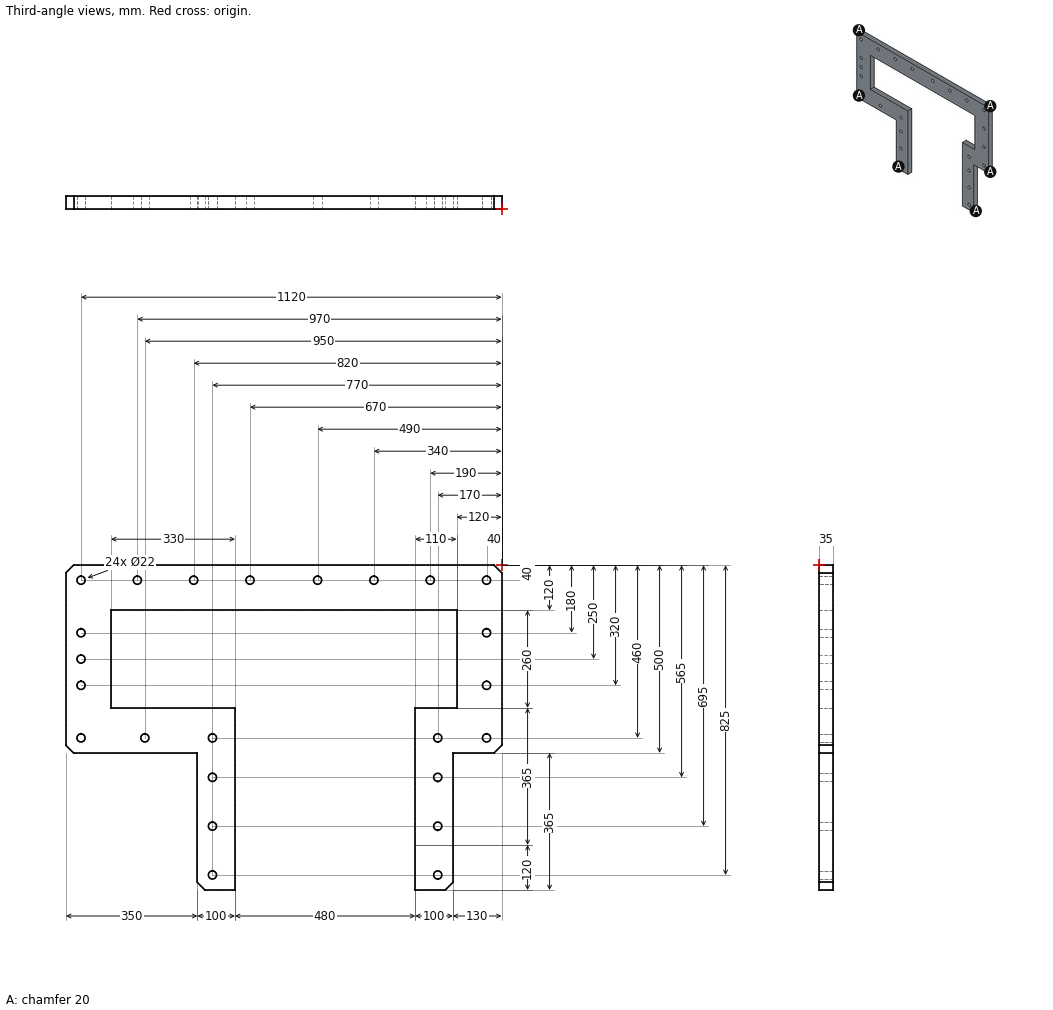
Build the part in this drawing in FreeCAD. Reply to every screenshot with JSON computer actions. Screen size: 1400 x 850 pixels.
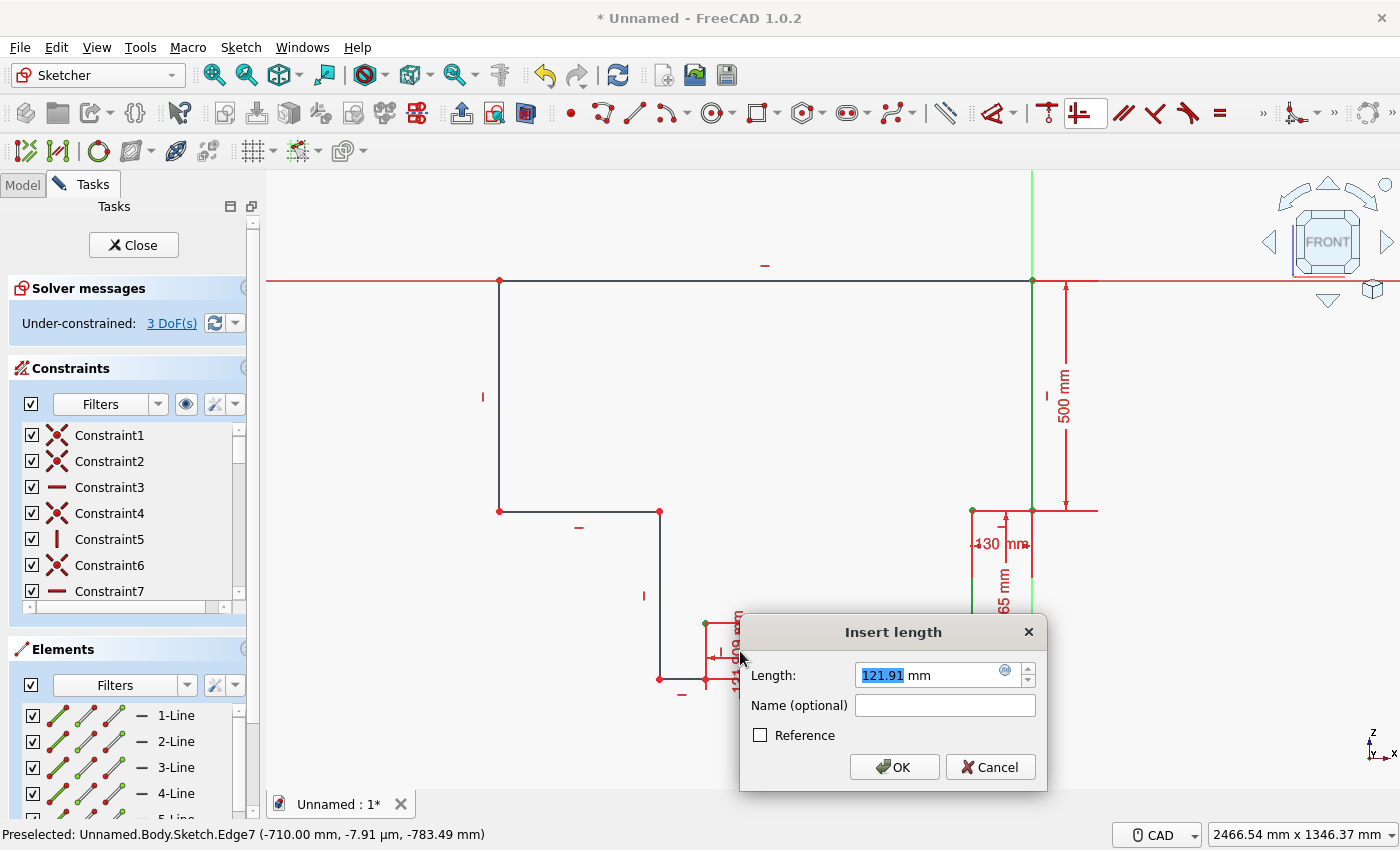
{"action": "type", "text": "120"}
{"action": "key", "text": "Return"}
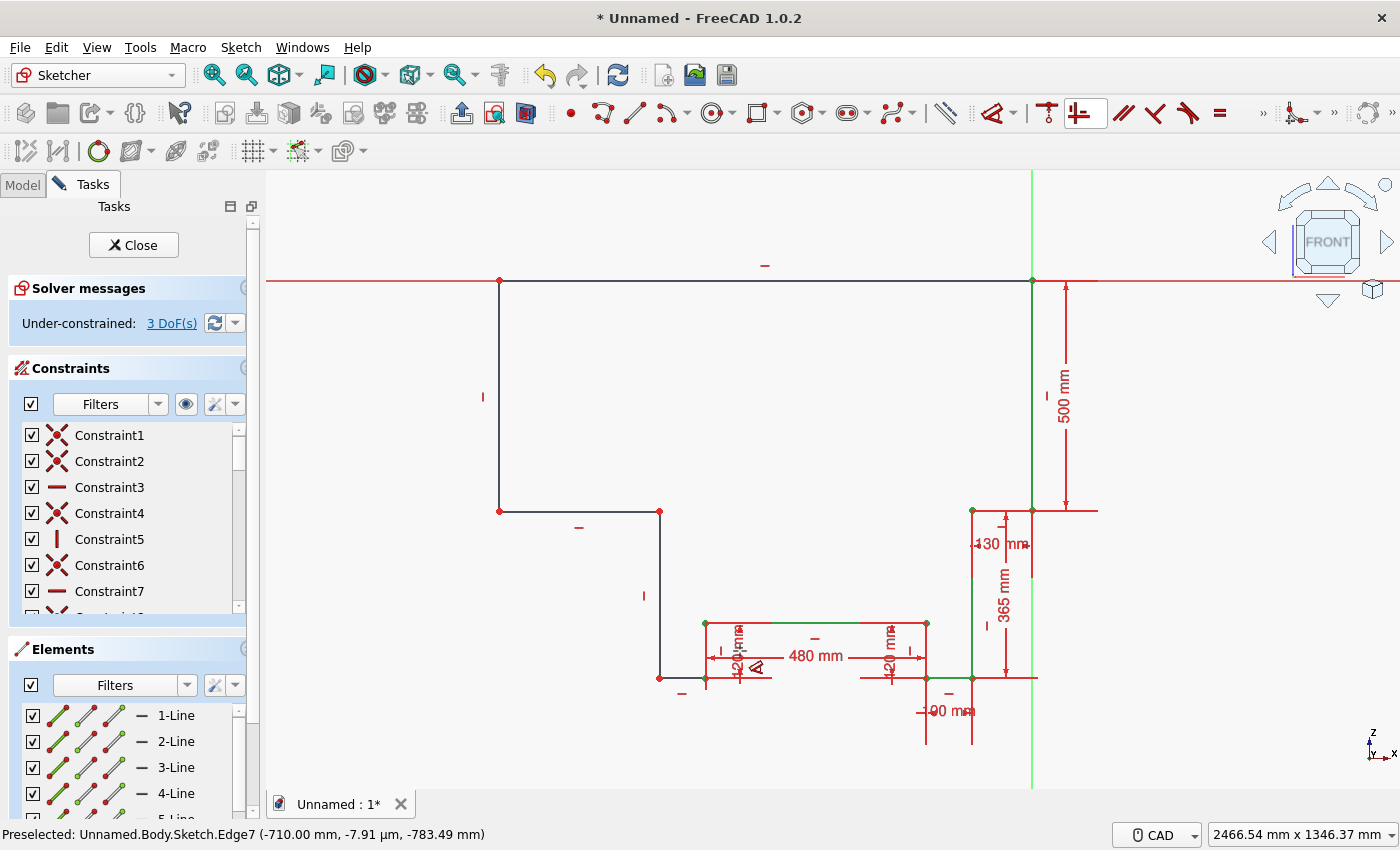
{"action": "left_click", "coordinate": [692, 678]}
{"action": "left_click", "coordinate": [683, 712]}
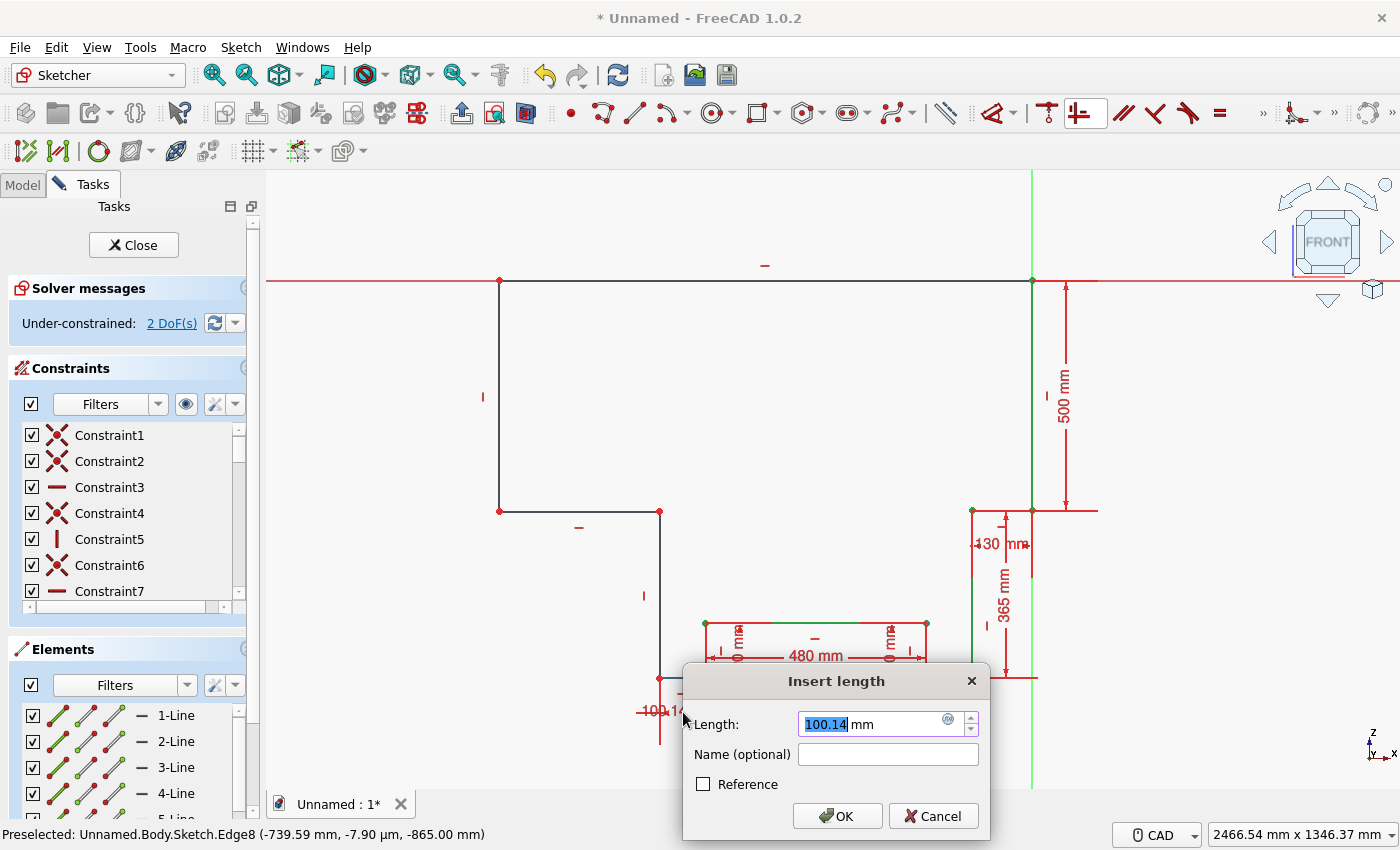
{"action": "type", "text": "100"}
{"action": "key", "text": "Return"}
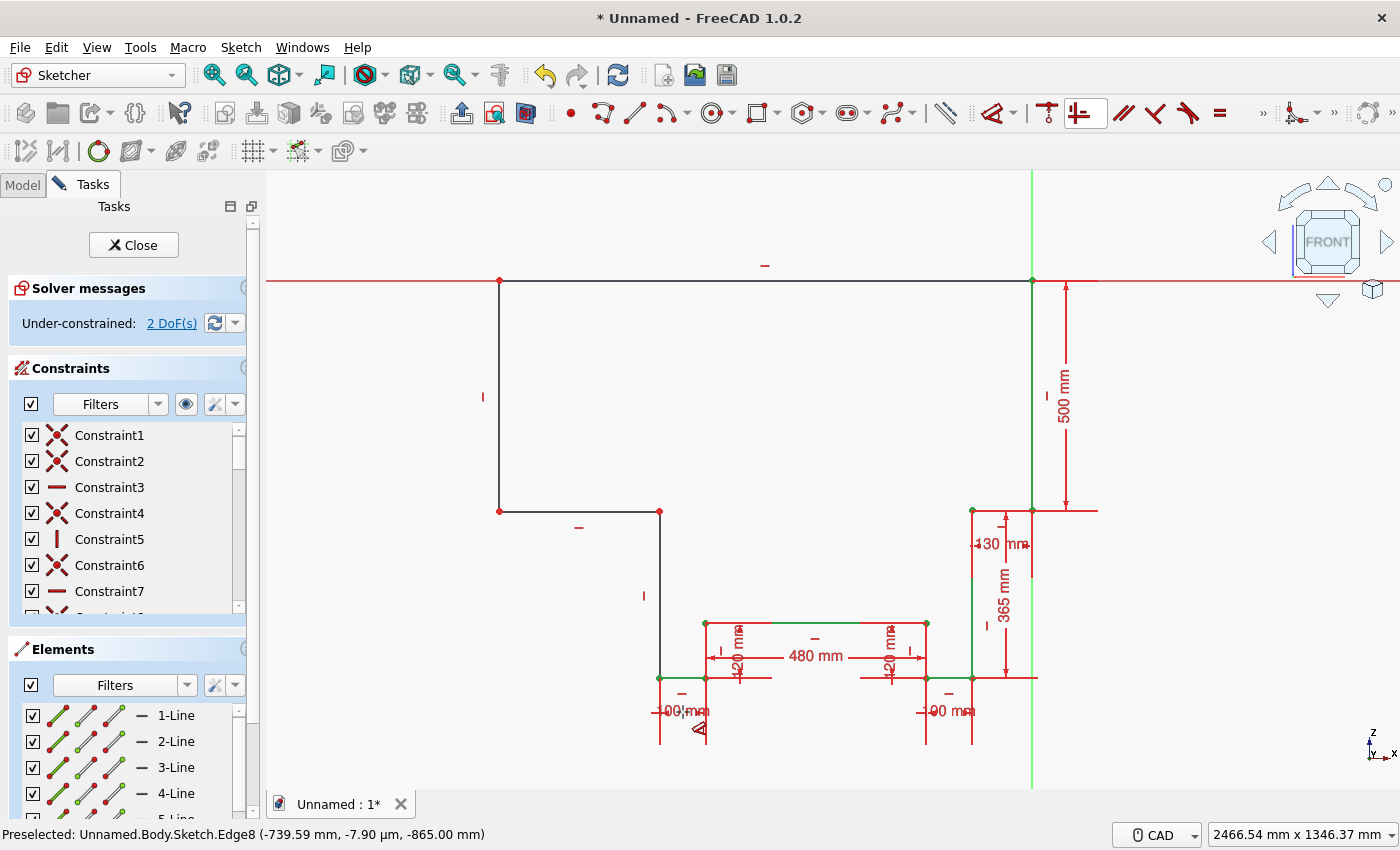
{"action": "left_click", "coordinate": [660, 629]}
{"action": "left_click", "coordinate": [626, 595]}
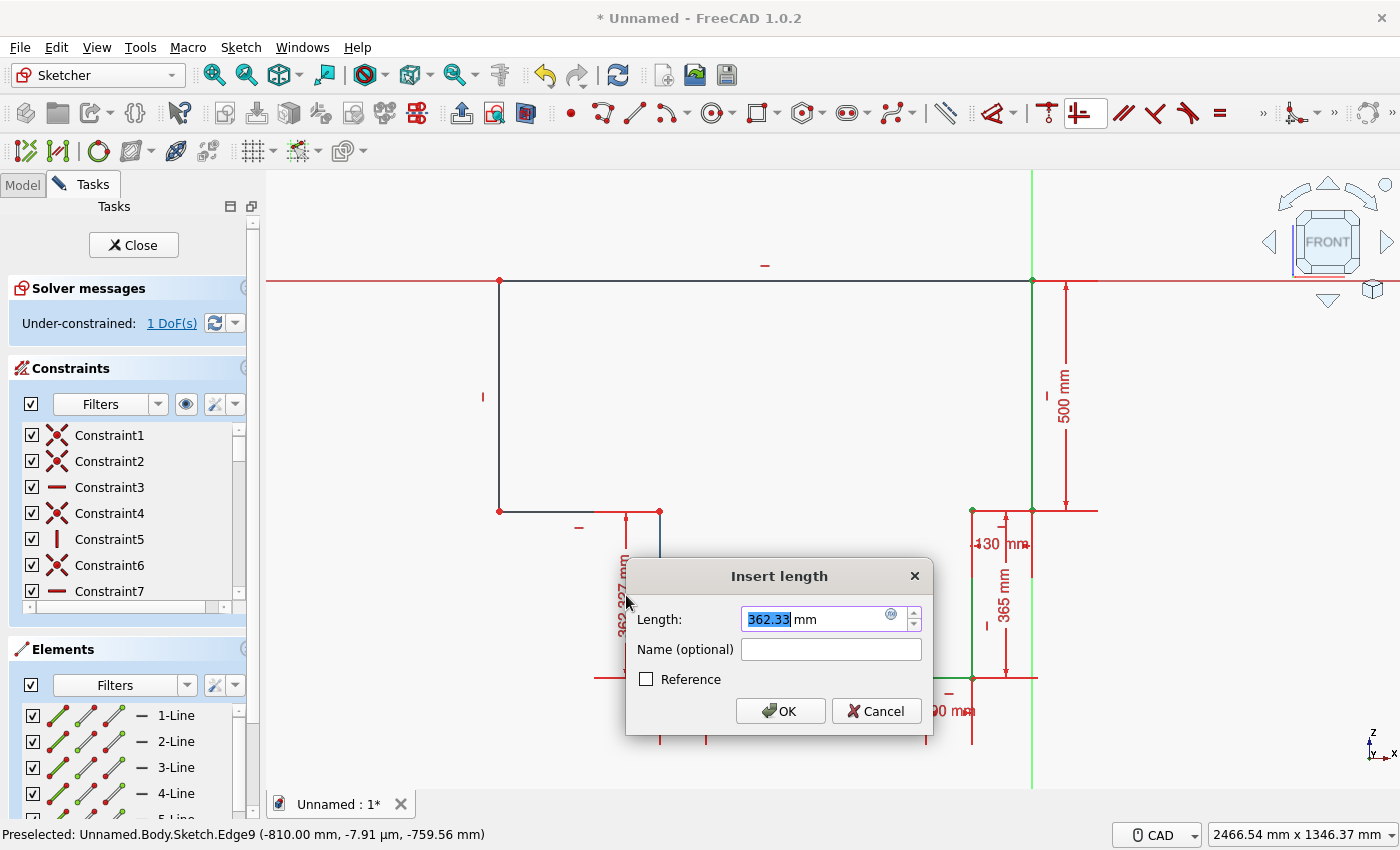
{"action": "type", "text": "365"}
{"action": "key", "text": "Return"}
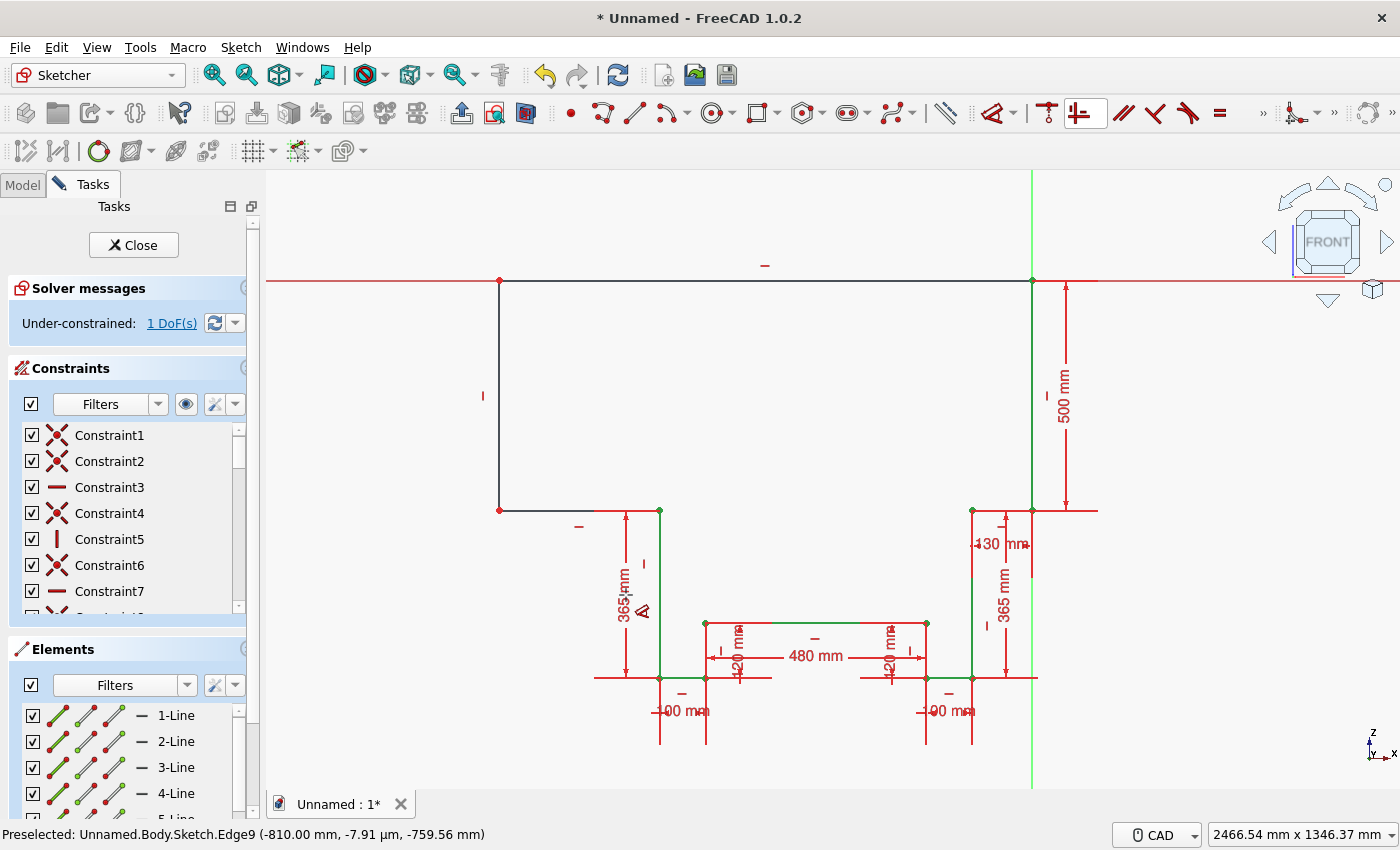
{"action": "left_click", "coordinate": [611, 511]}
{"action": "left_click", "coordinate": [579, 545]}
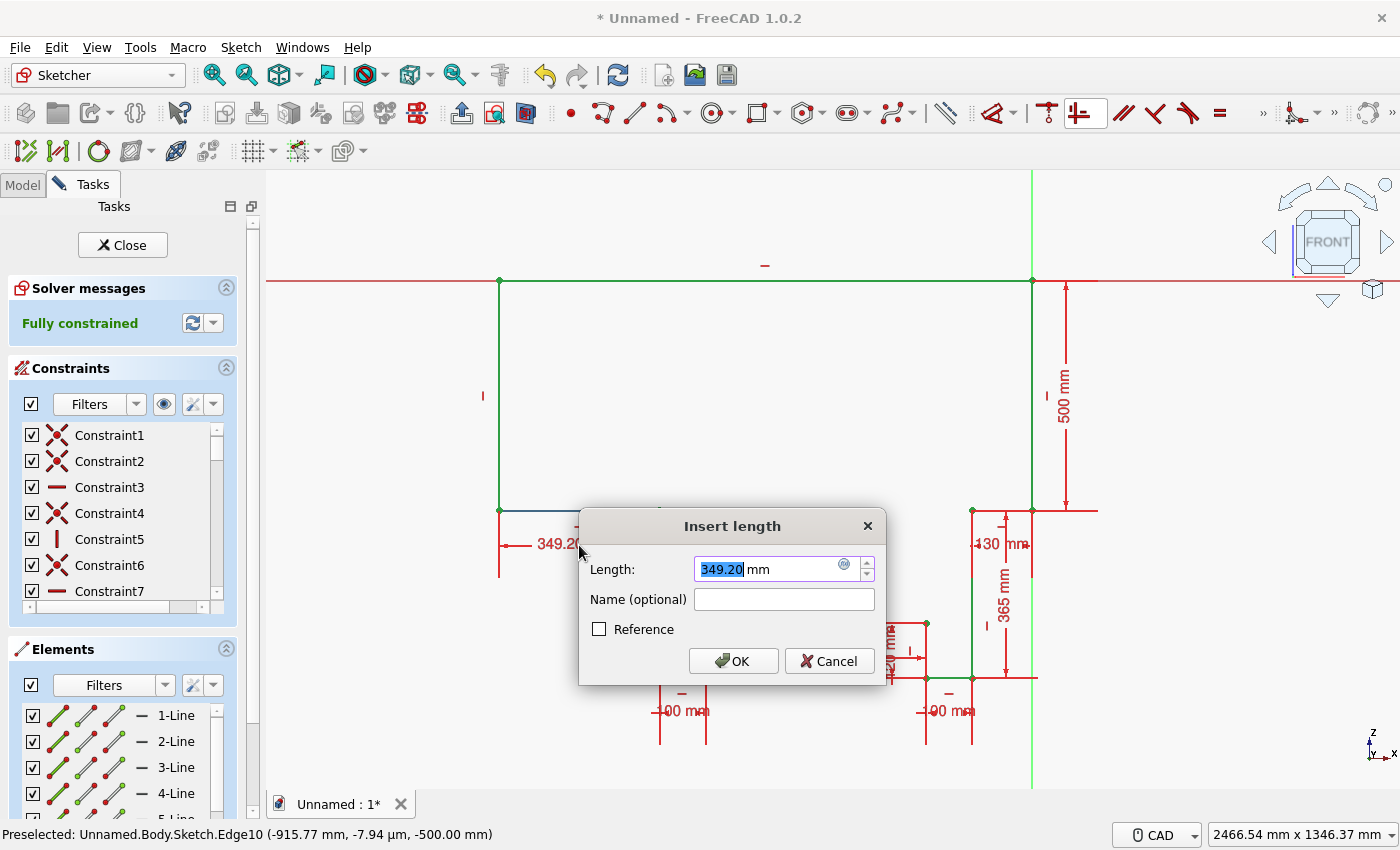
{"action": "type", "text": "350"}
{"action": "key", "text": "Return"}
{"action": "key", "text": "Escape"}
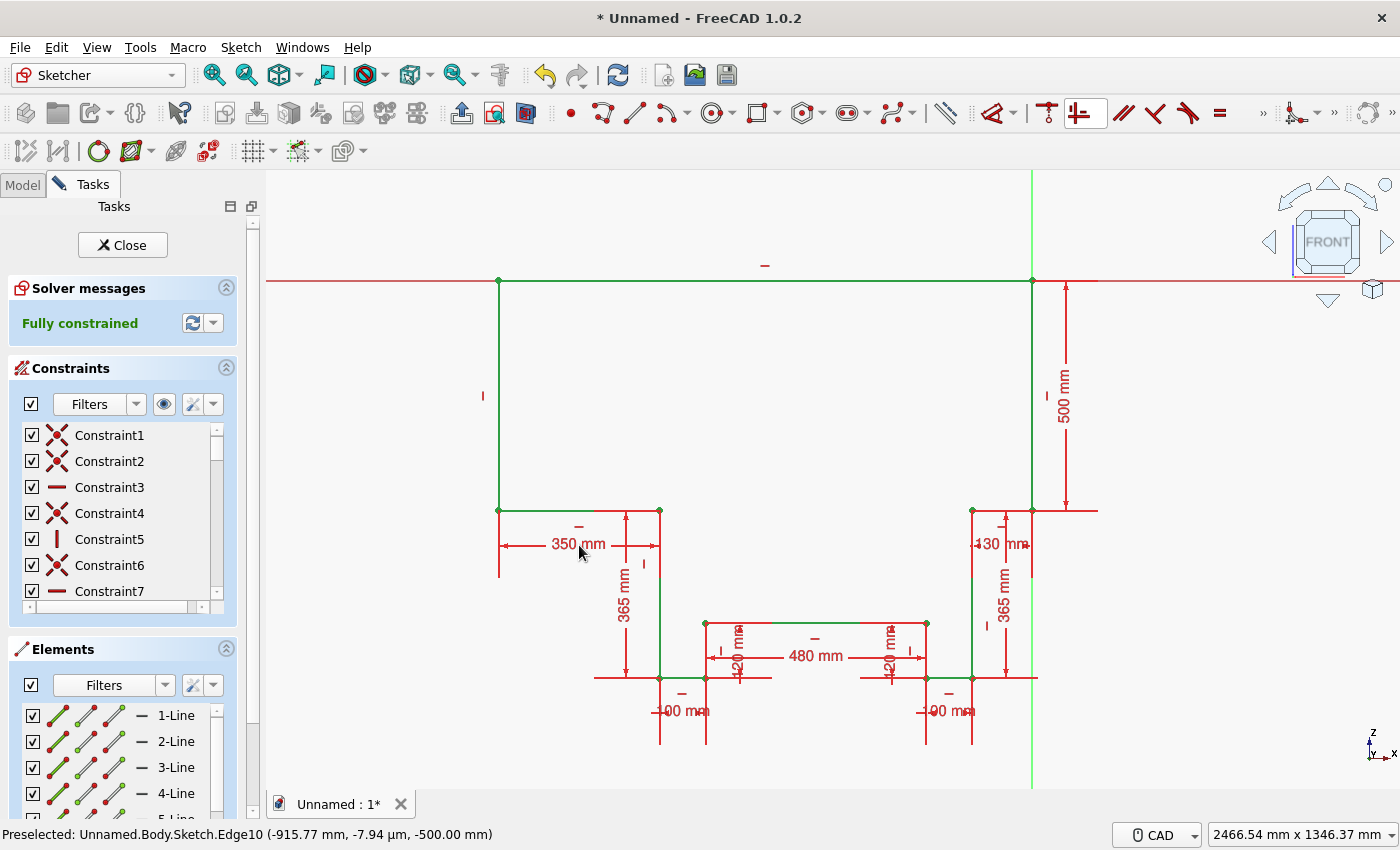
{"action": "left_click", "coordinate": [123, 245]}